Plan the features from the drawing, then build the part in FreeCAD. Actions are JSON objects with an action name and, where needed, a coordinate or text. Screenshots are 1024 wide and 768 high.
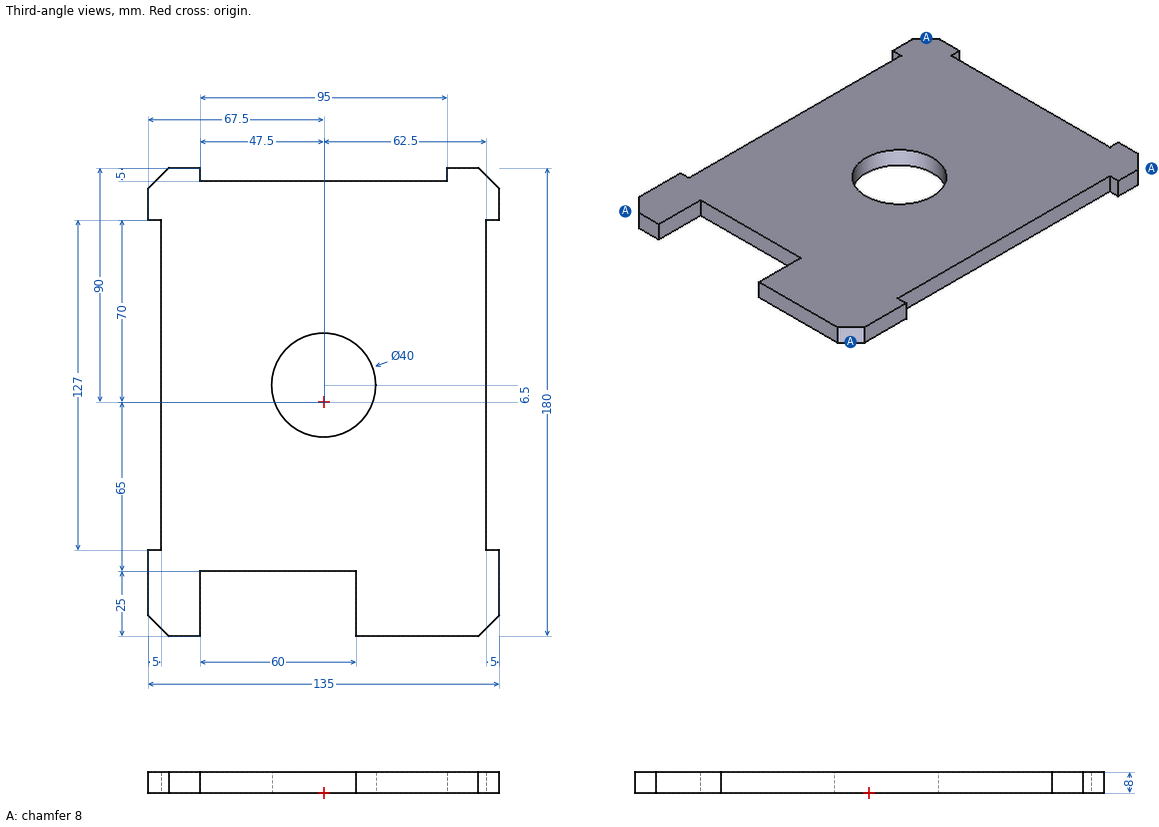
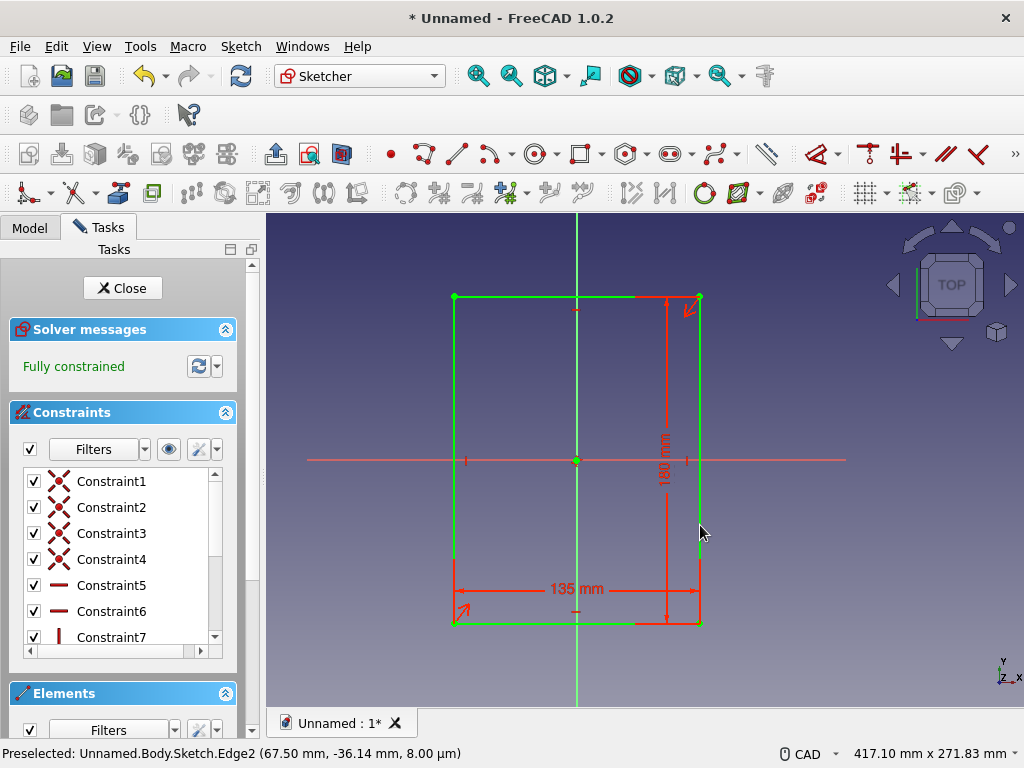
{"action": "left_click", "coordinate": [123, 288]}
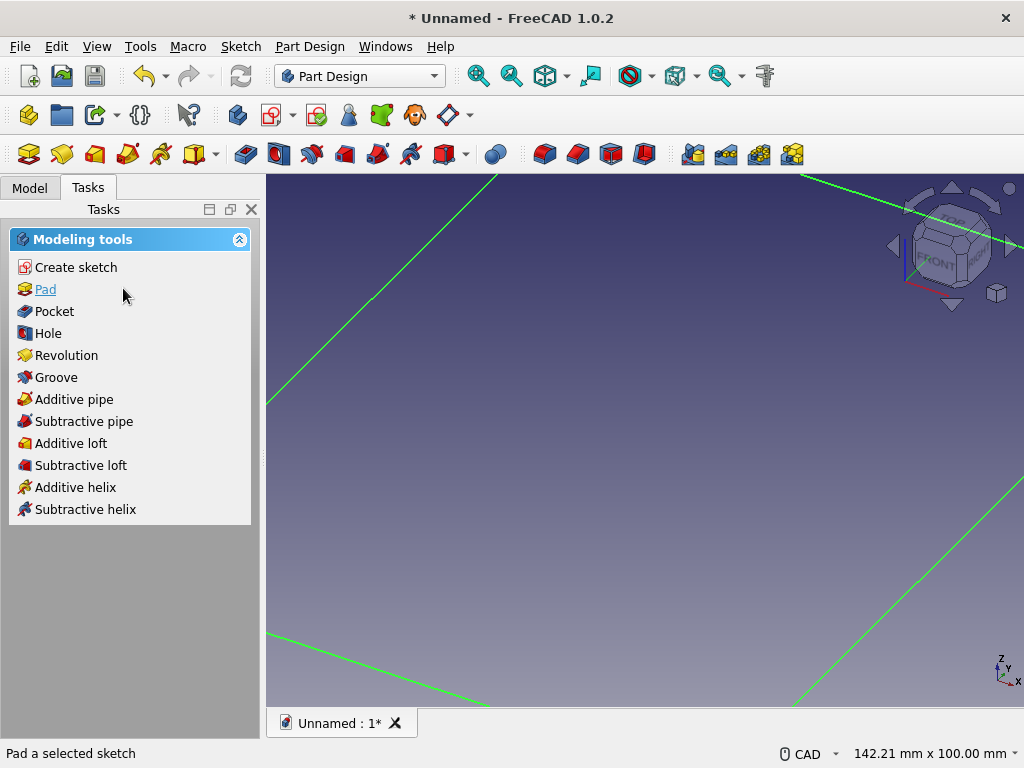
{"action": "left_click", "coordinate": [29, 154]}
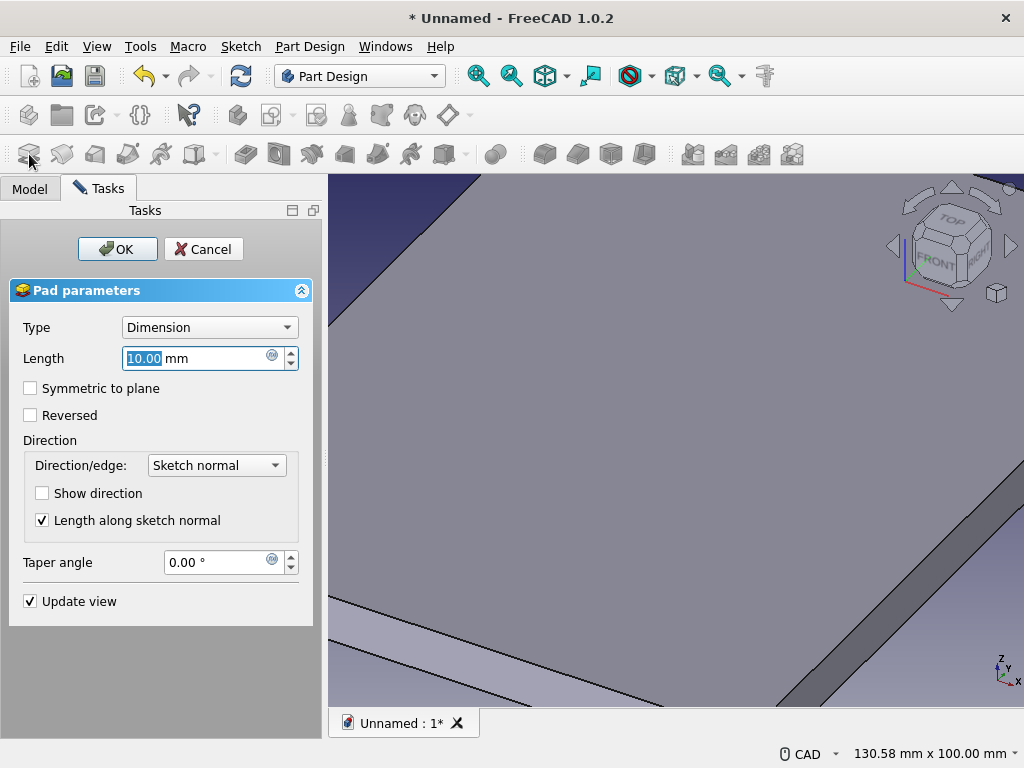
{"action": "type", "text": "8"}
{"action": "key", "text": "Tab"}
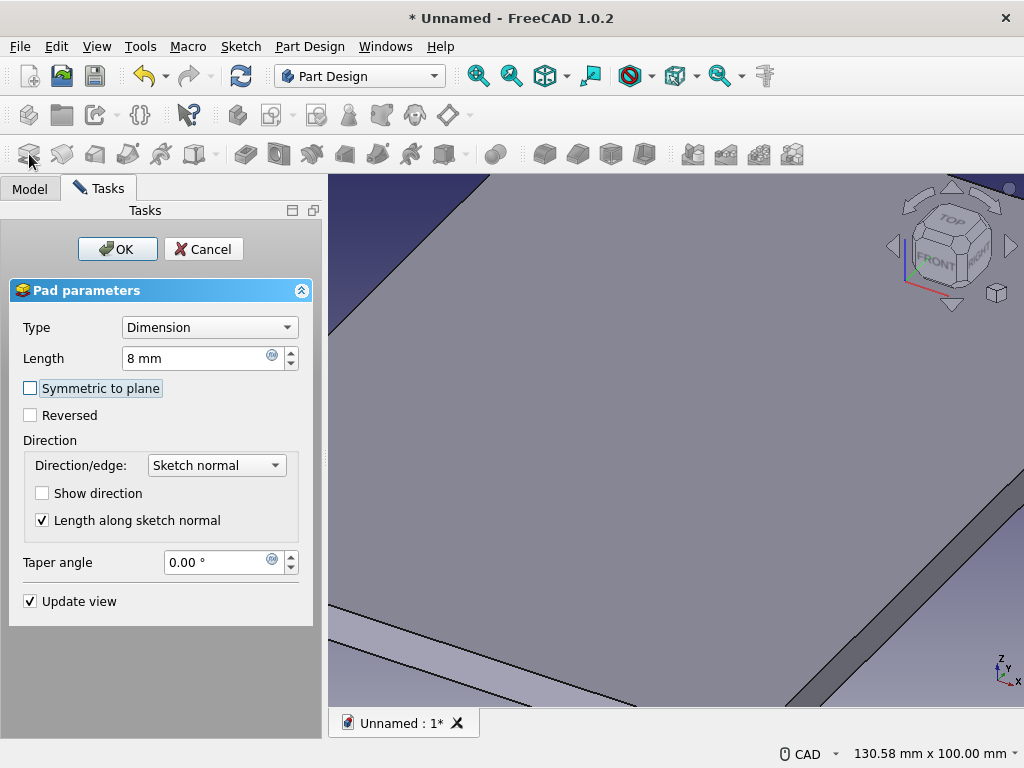
{"action": "left_click", "coordinate": [118, 249]}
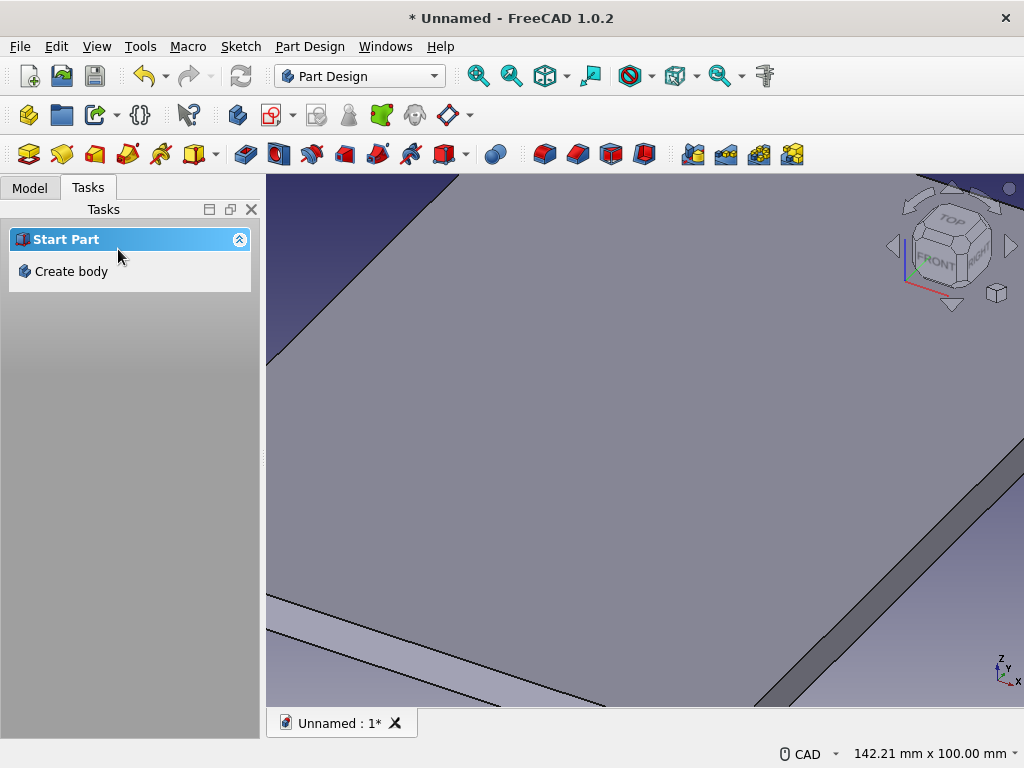
{"action": "key", "text": "v f"}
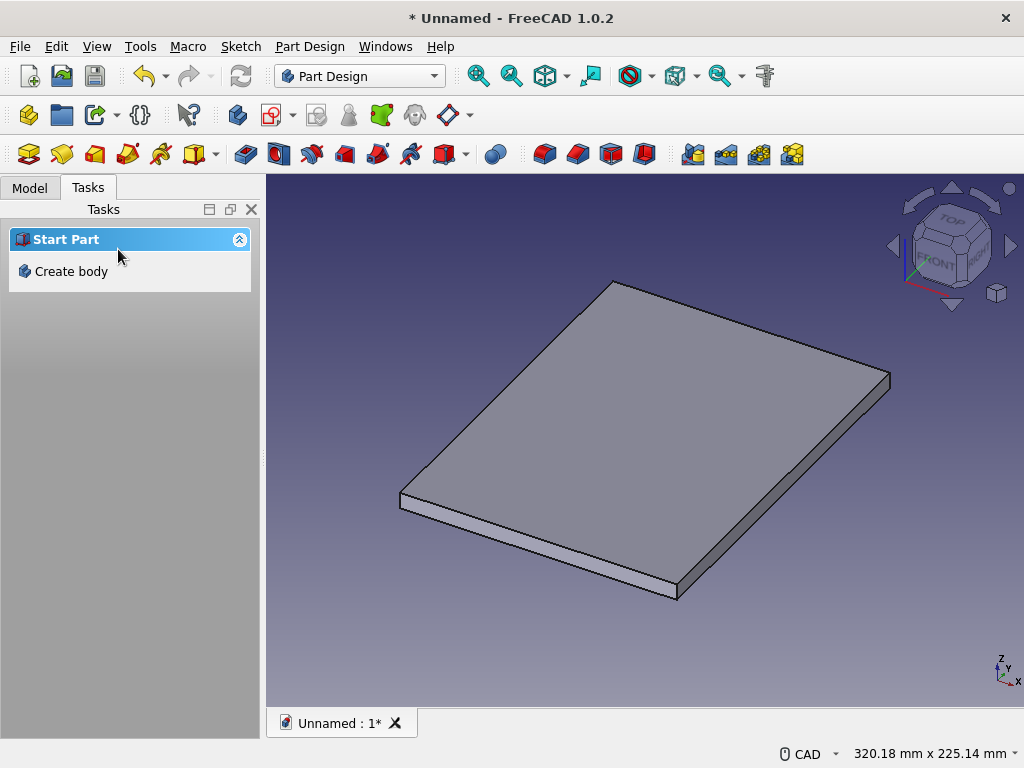
{"action": "left_click", "coordinate": [645, 432]}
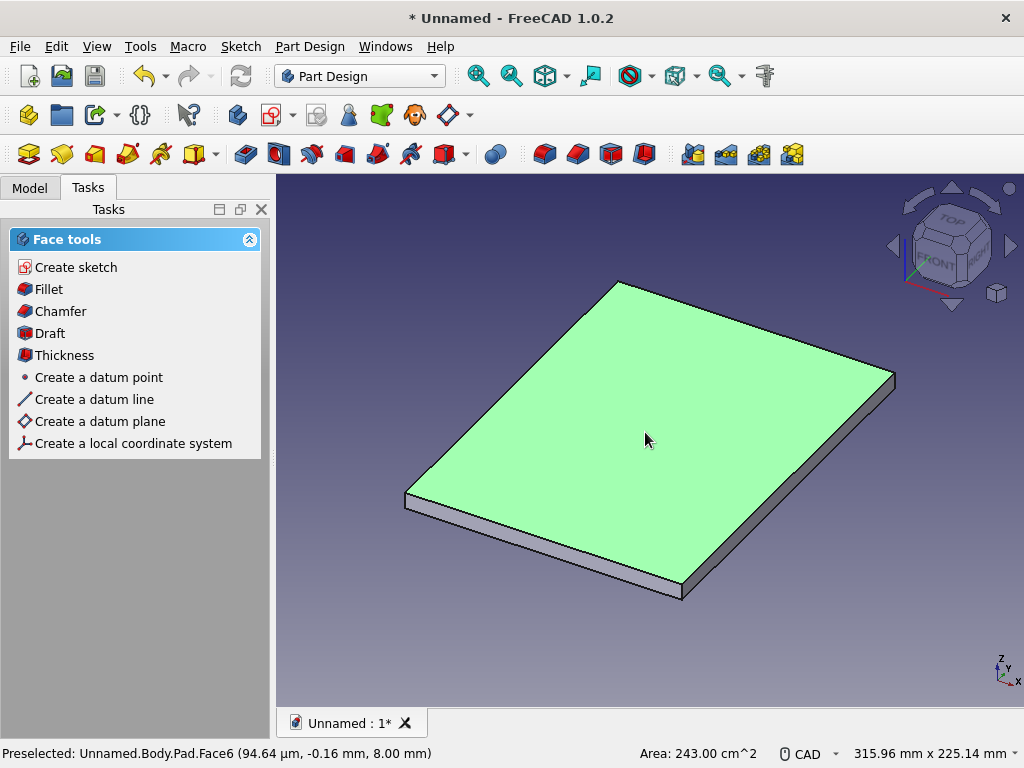
{"action": "left_click", "coordinate": [270, 116]}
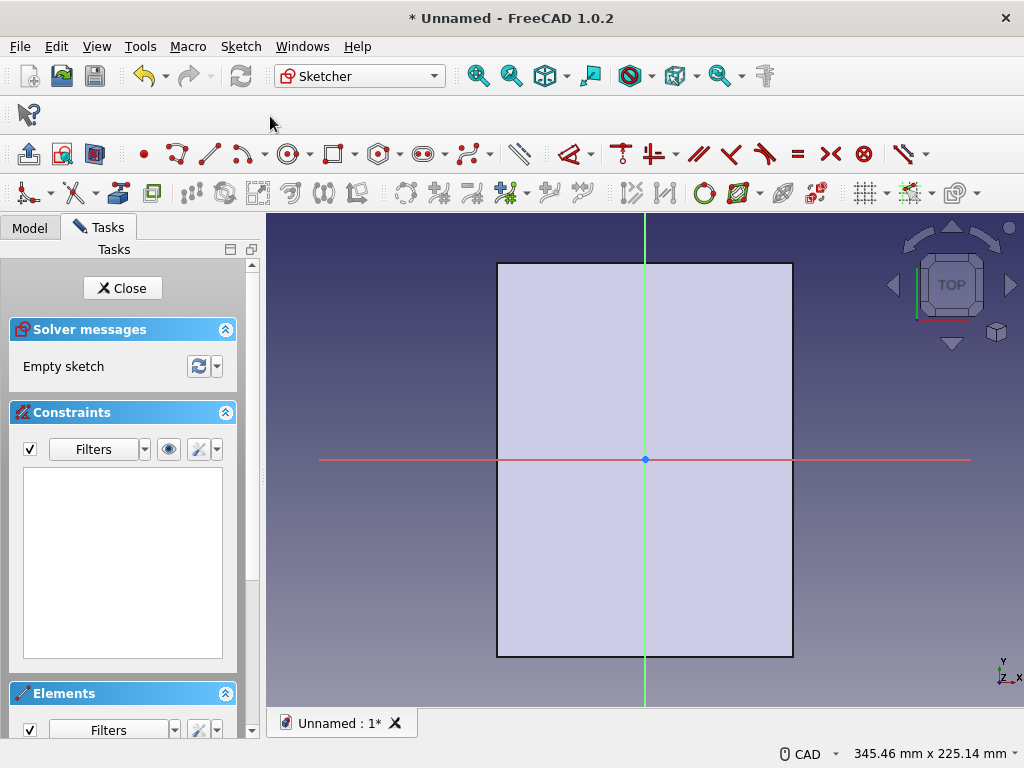
{"action": "scroll", "coordinate": [784, 241], "scroll_direction": "up", "scroll_amount": 2}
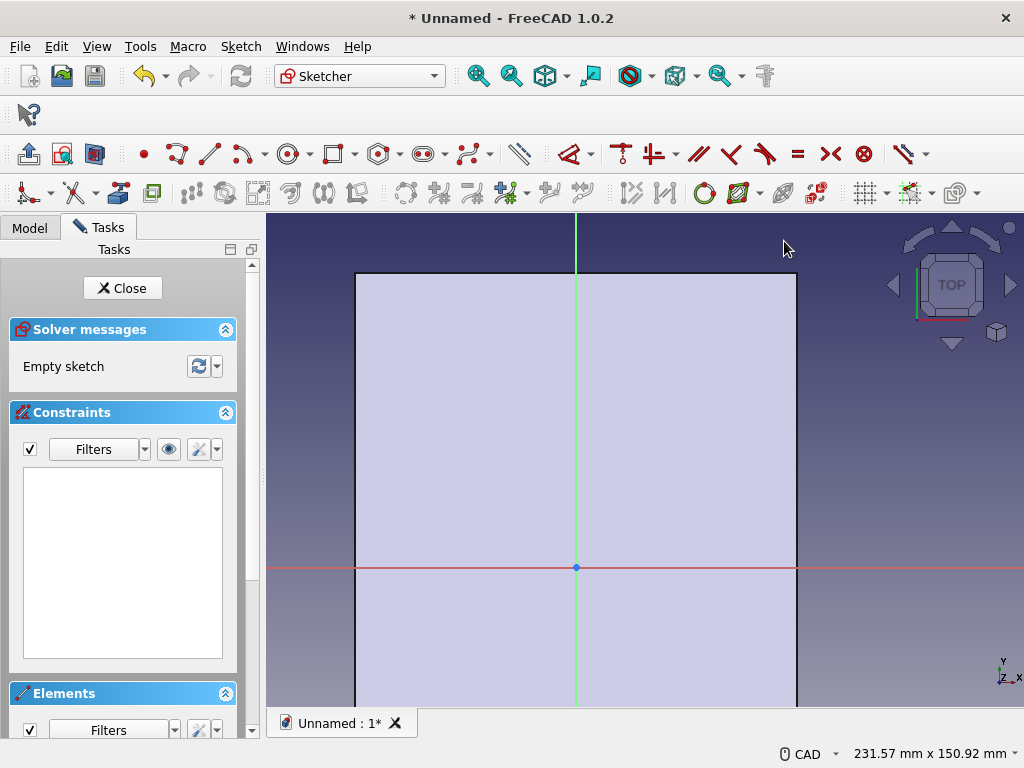
{"action": "key", "text": "g r"}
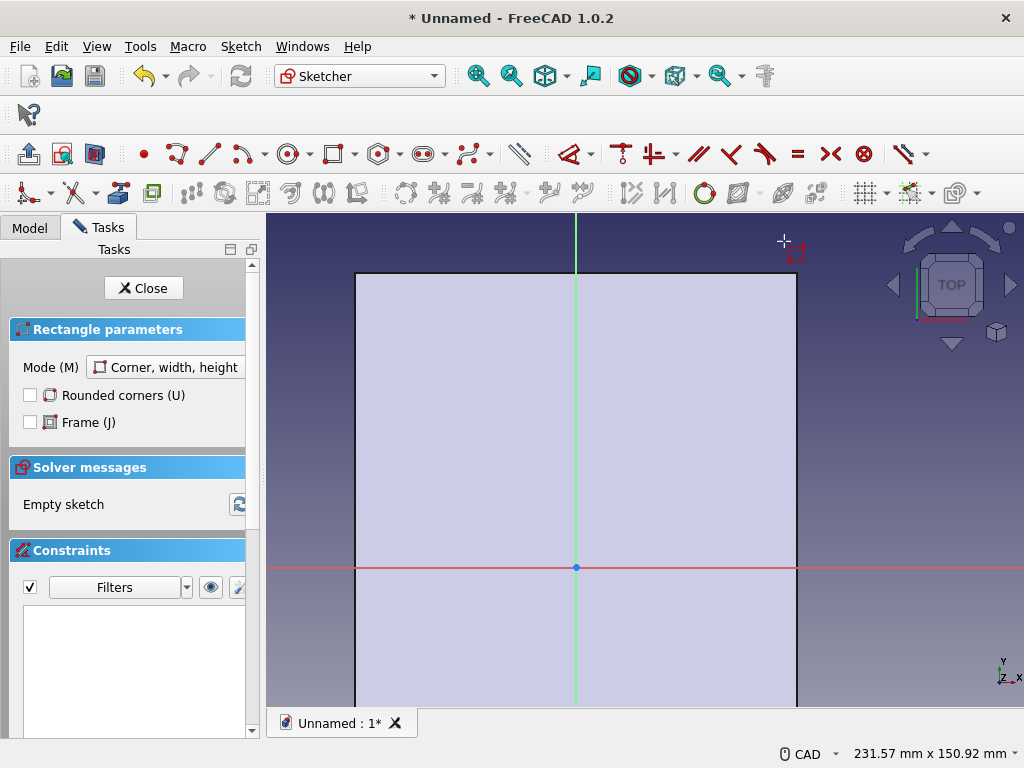
{"action": "left_click", "coordinate": [421, 273]}
{"action": "left_click", "coordinate": [732, 289]}
{"action": "key", "text": "Escape"}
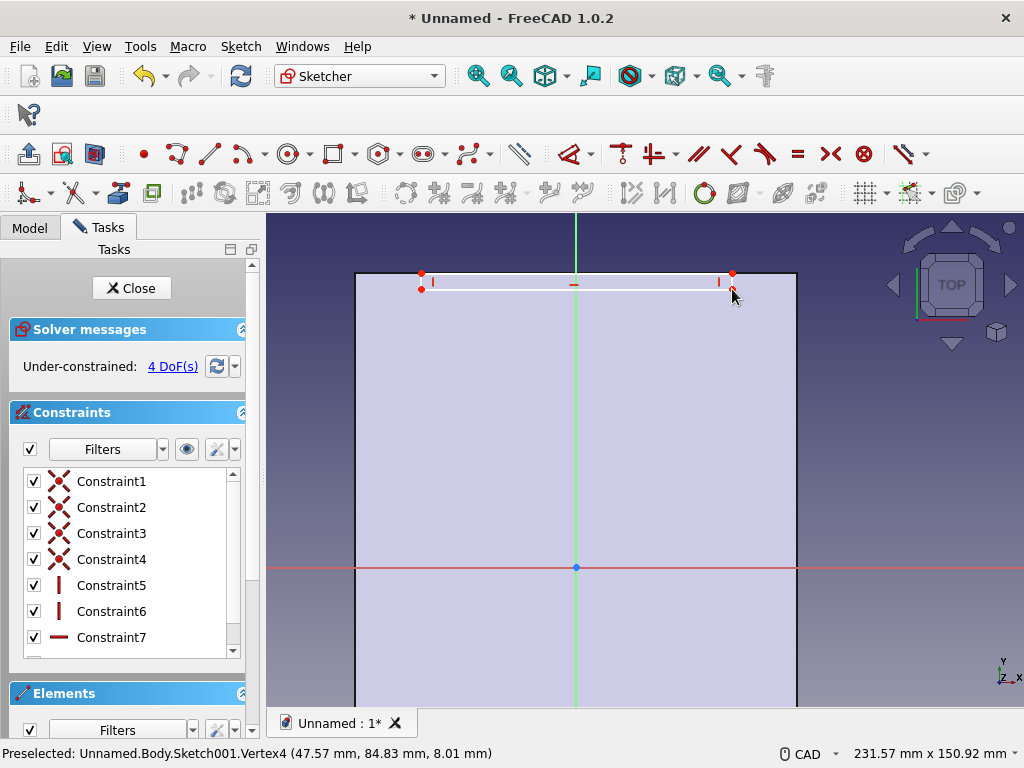
{"action": "scroll", "coordinate": [421, 282], "scroll_direction": "up", "scroll_amount": 5}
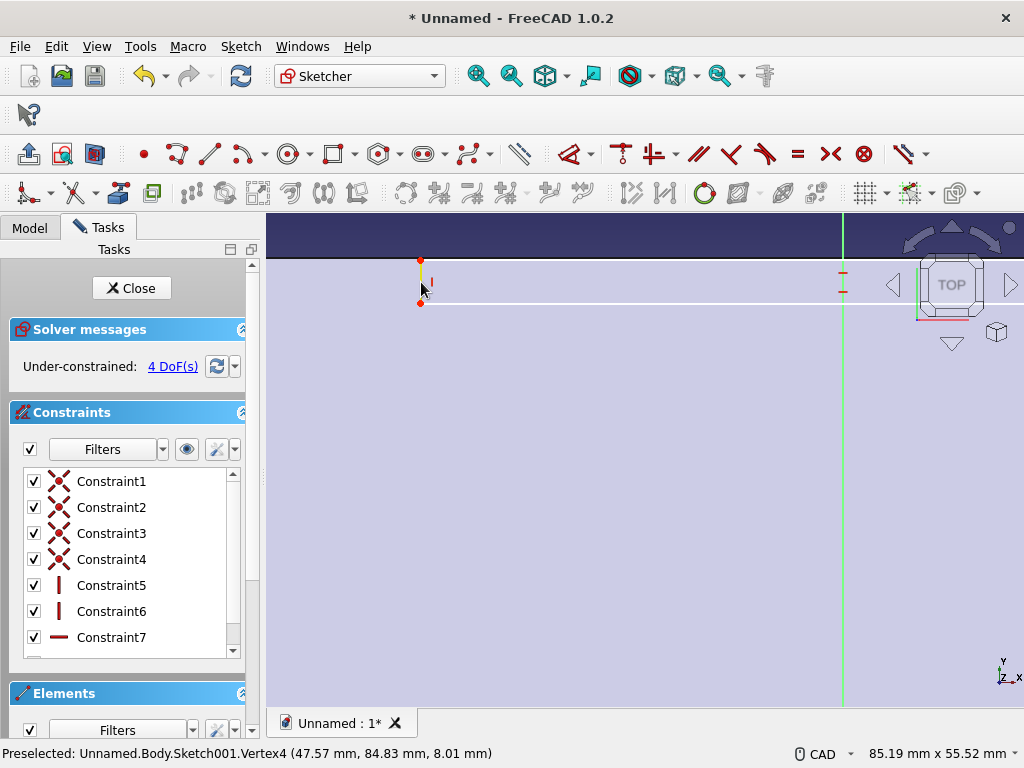
{"action": "left_click", "coordinate": [421, 282]}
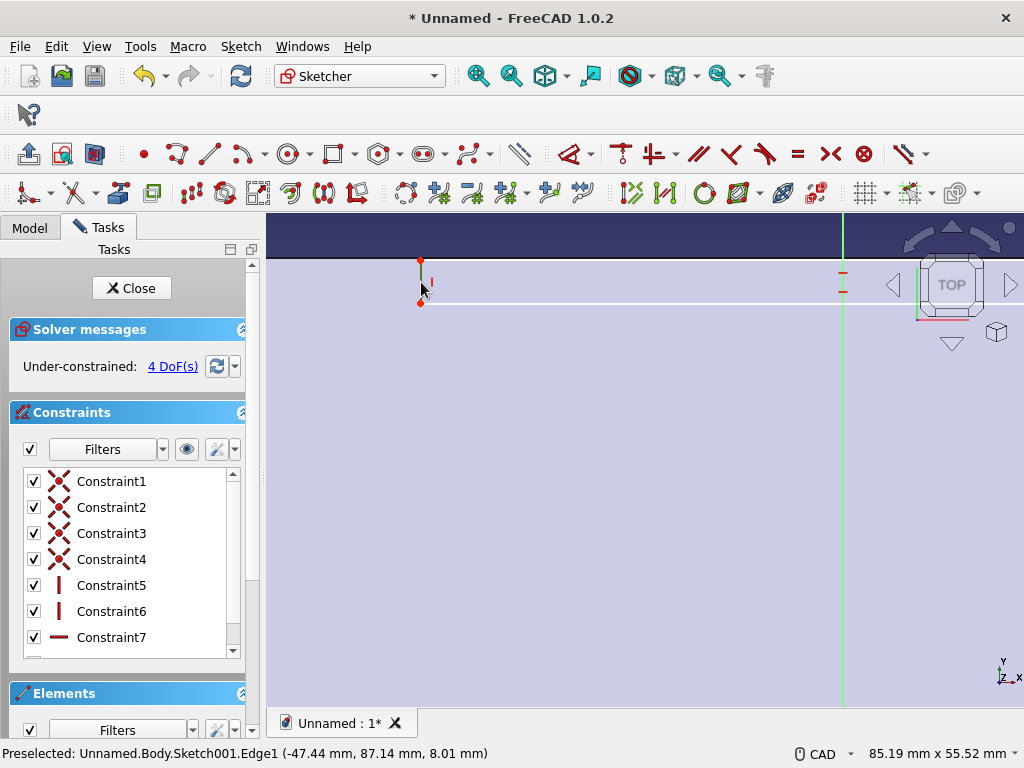
{"action": "key", "text": "i"}